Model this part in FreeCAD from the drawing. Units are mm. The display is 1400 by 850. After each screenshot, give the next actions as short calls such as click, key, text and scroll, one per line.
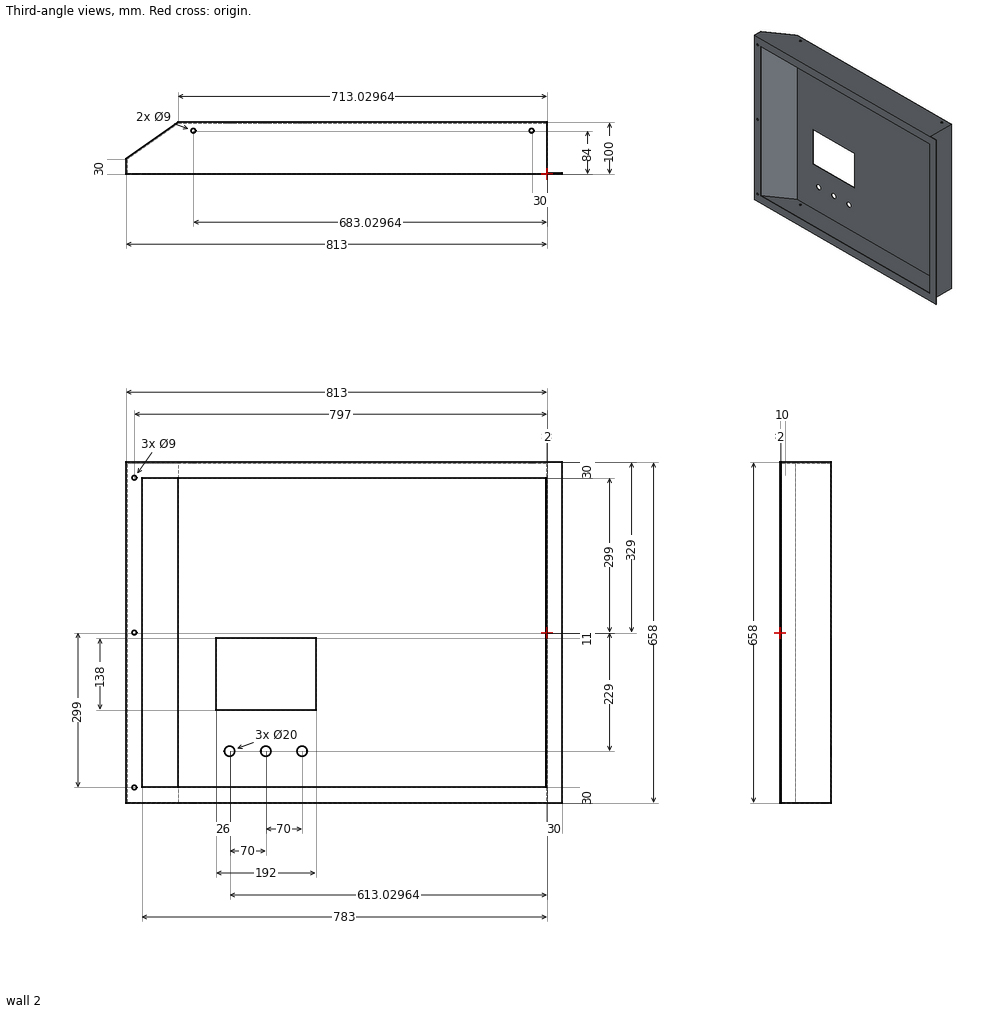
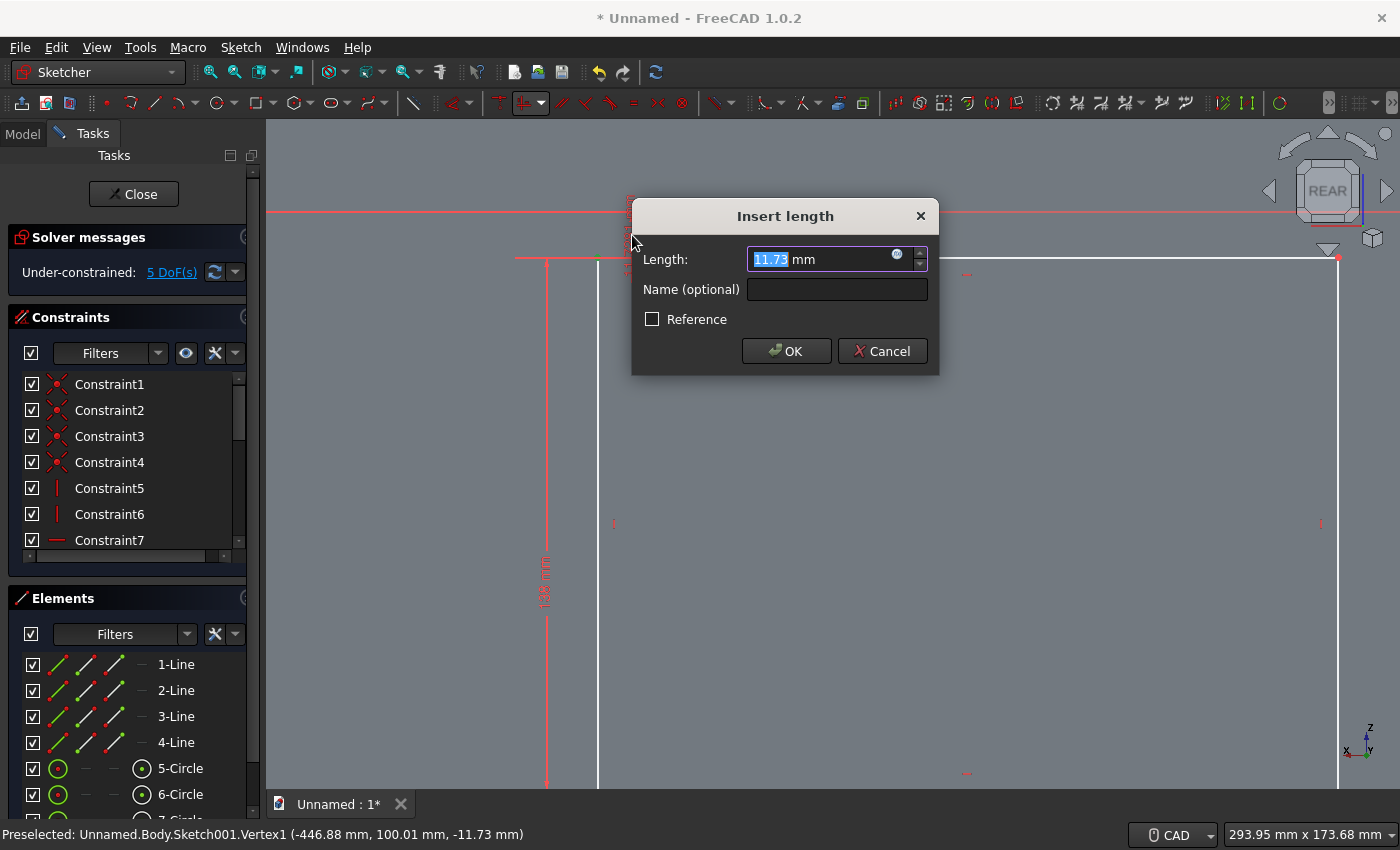
text(11)
key(Return)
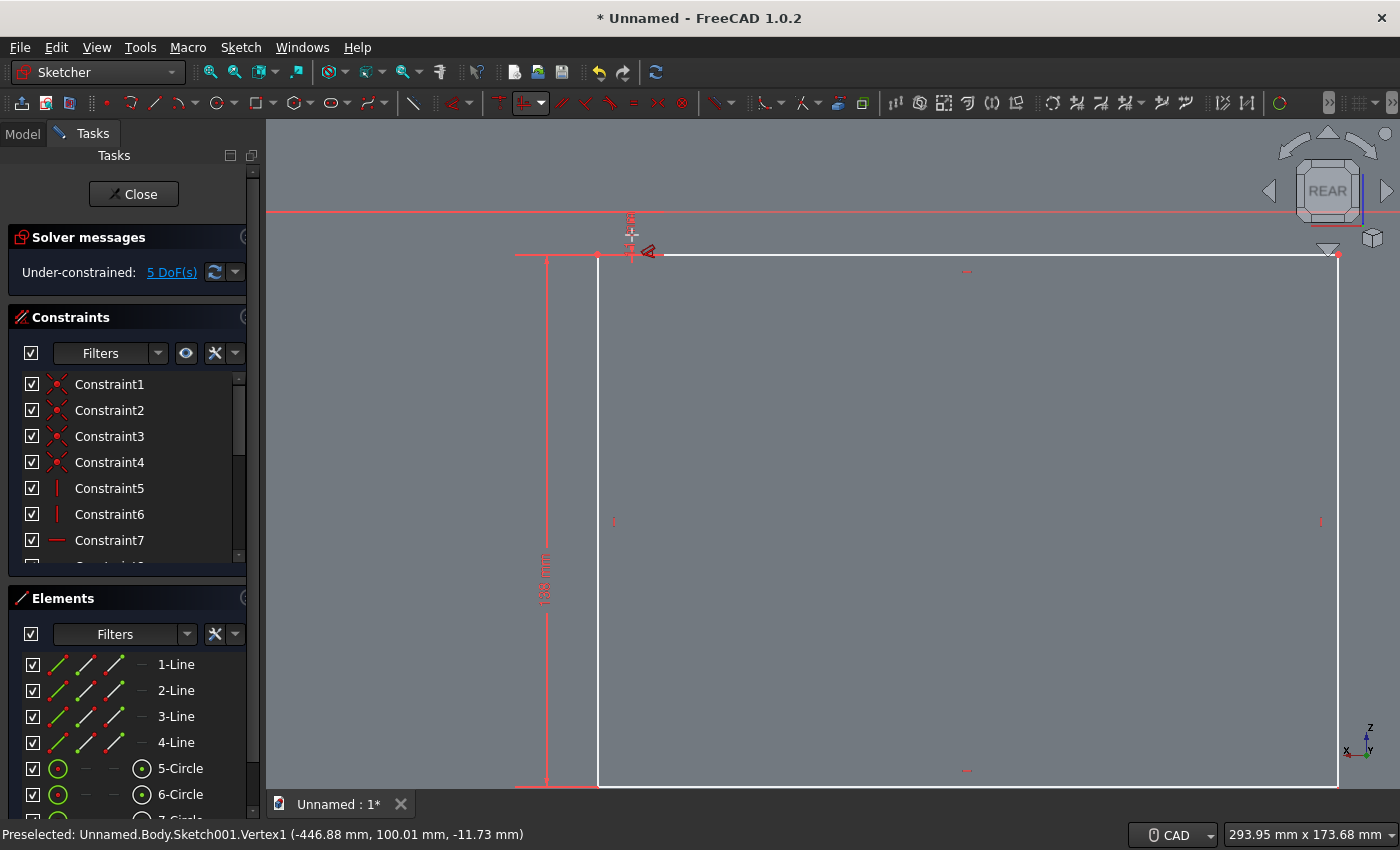
scroll(598, 258, down, 4)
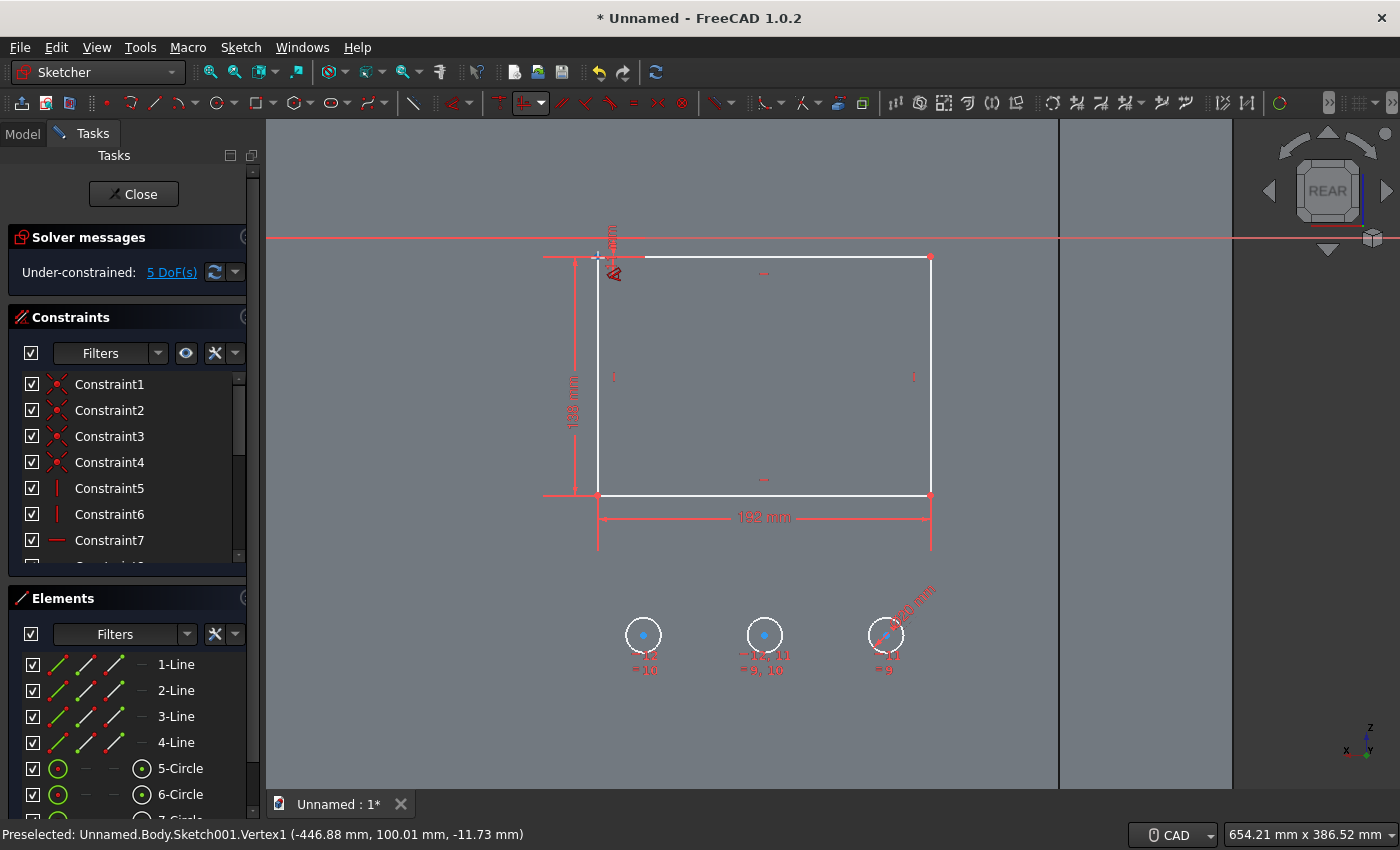
click(886, 635)
click(920, 528)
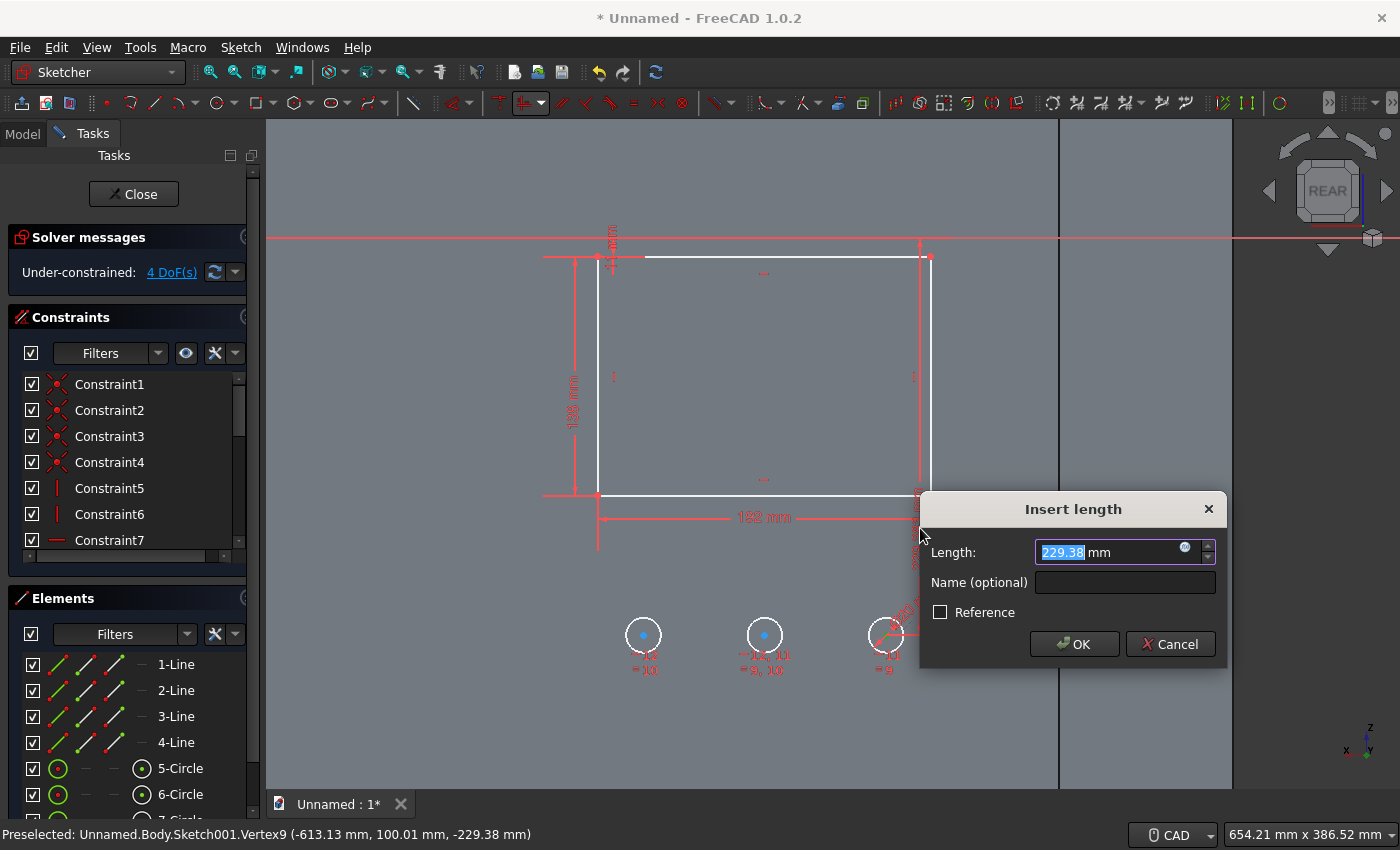
text(229)
key(Return)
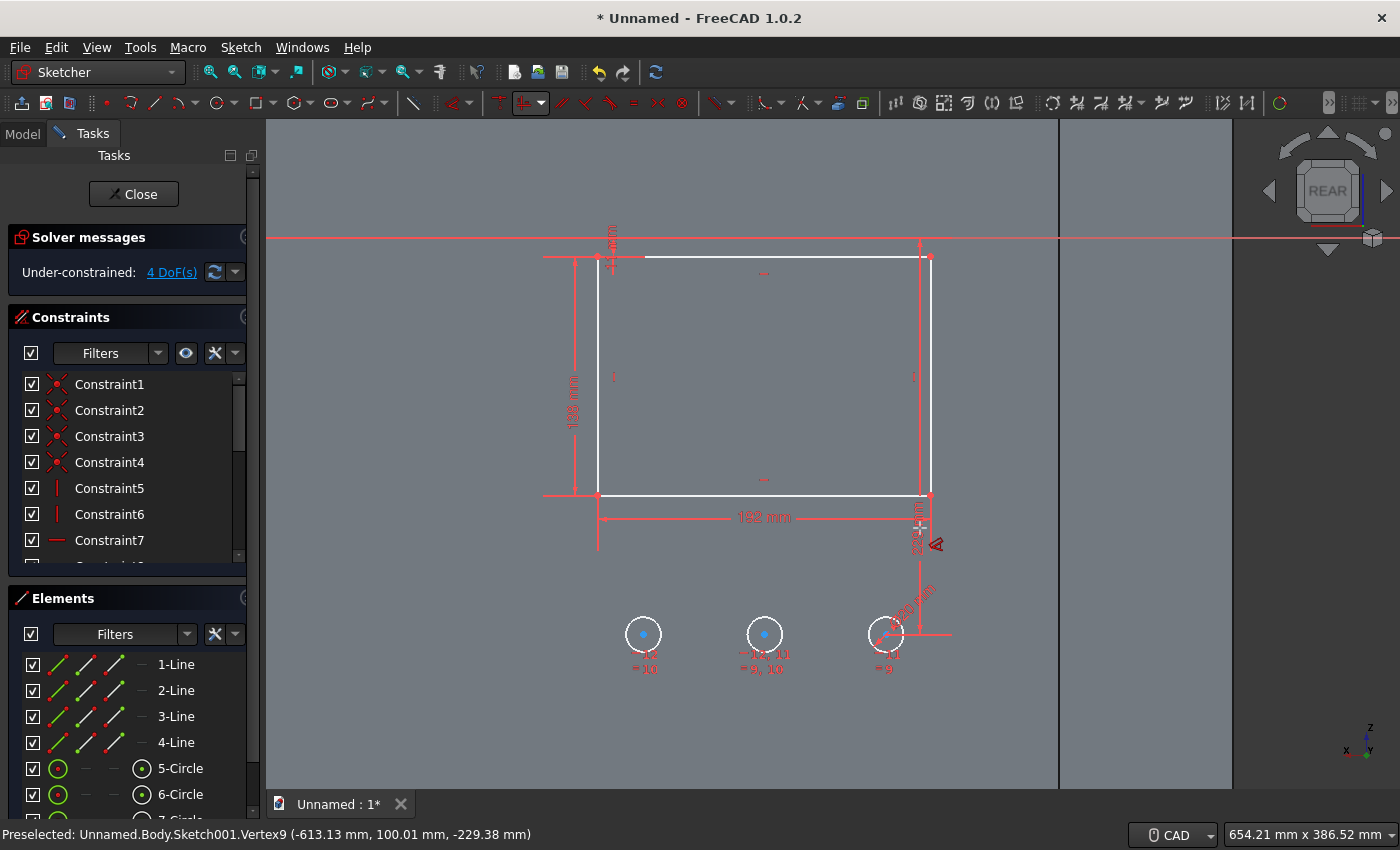
click(931, 496)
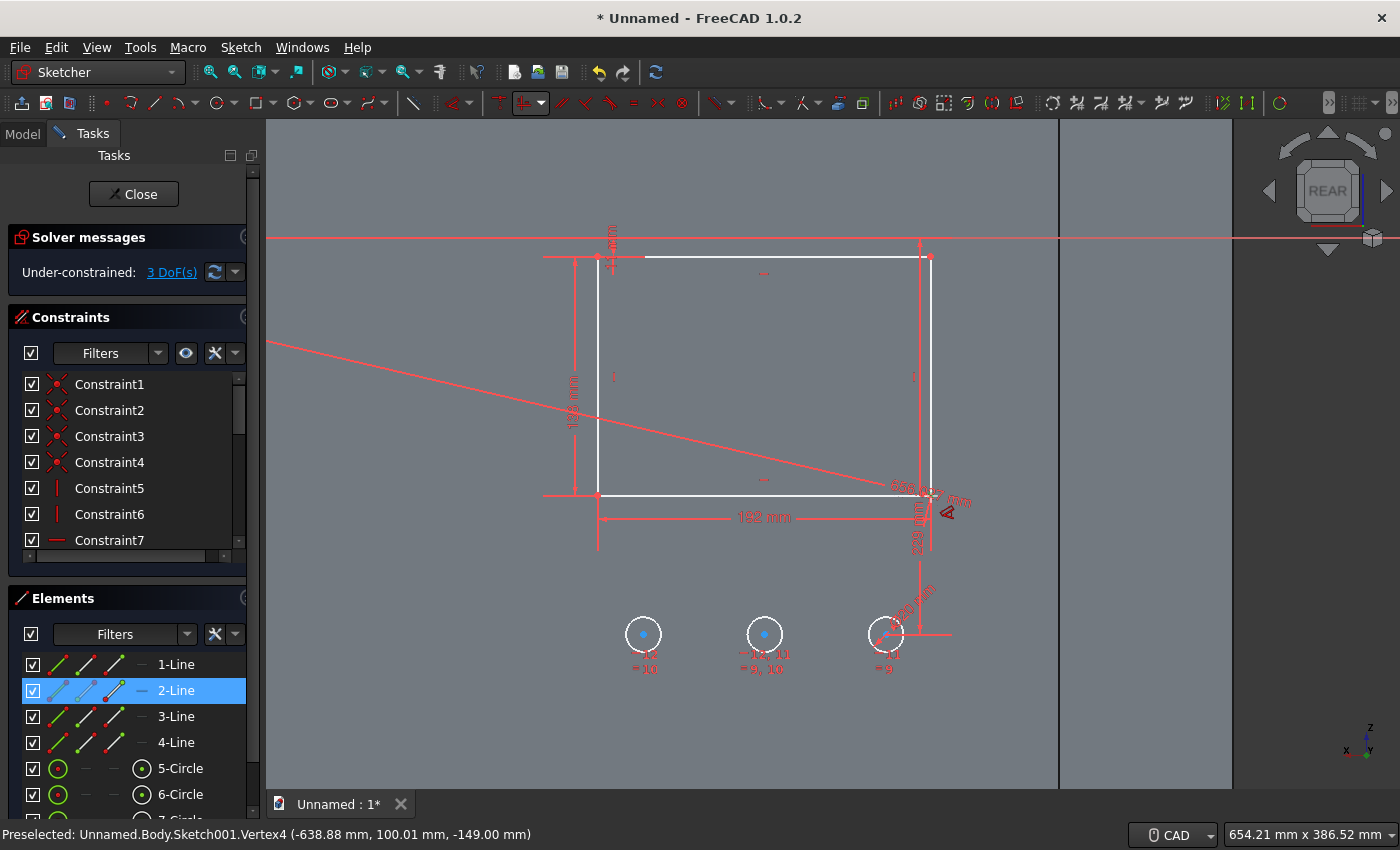
click(886, 635)
click(908, 669)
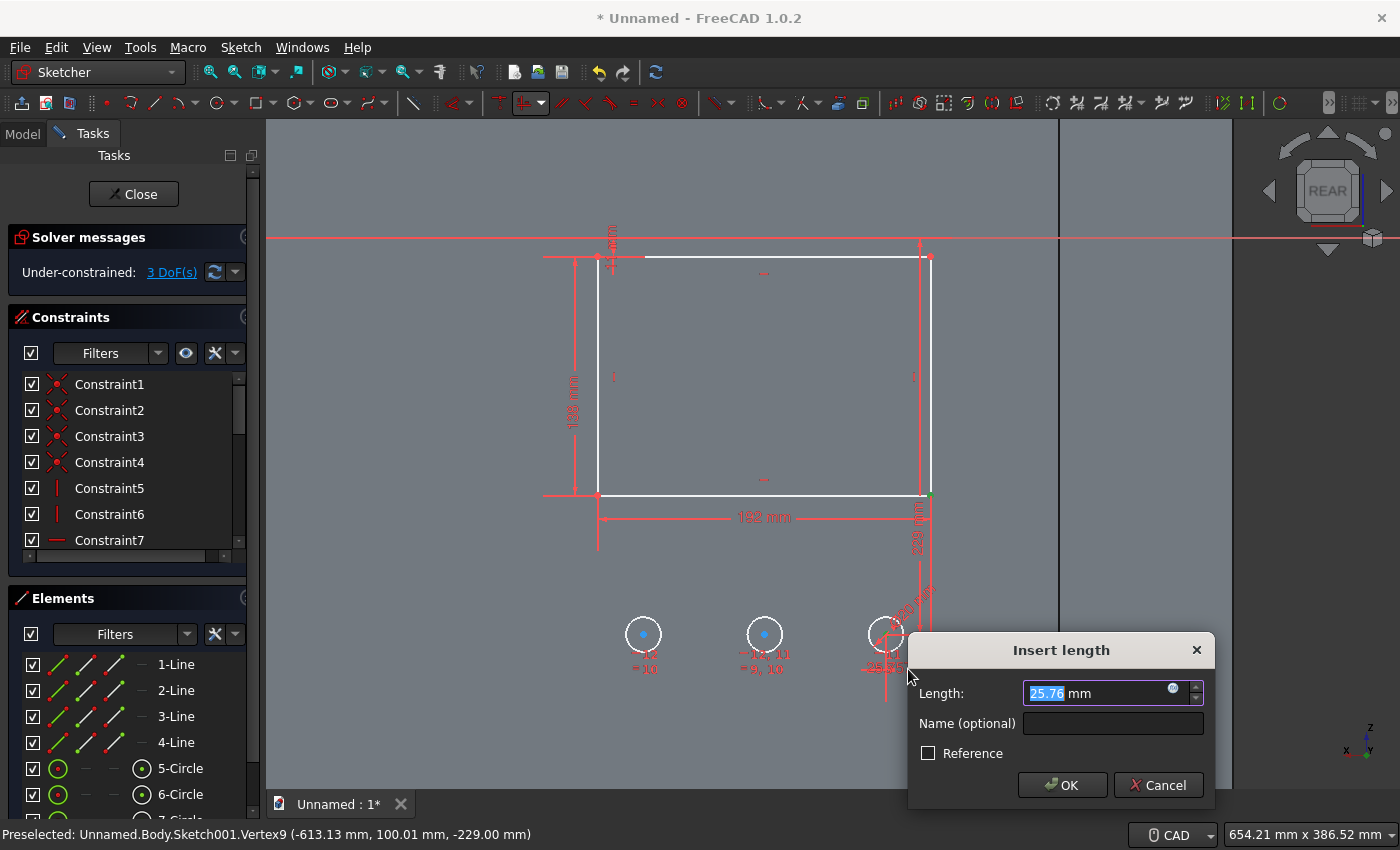
text(26)
key(Return)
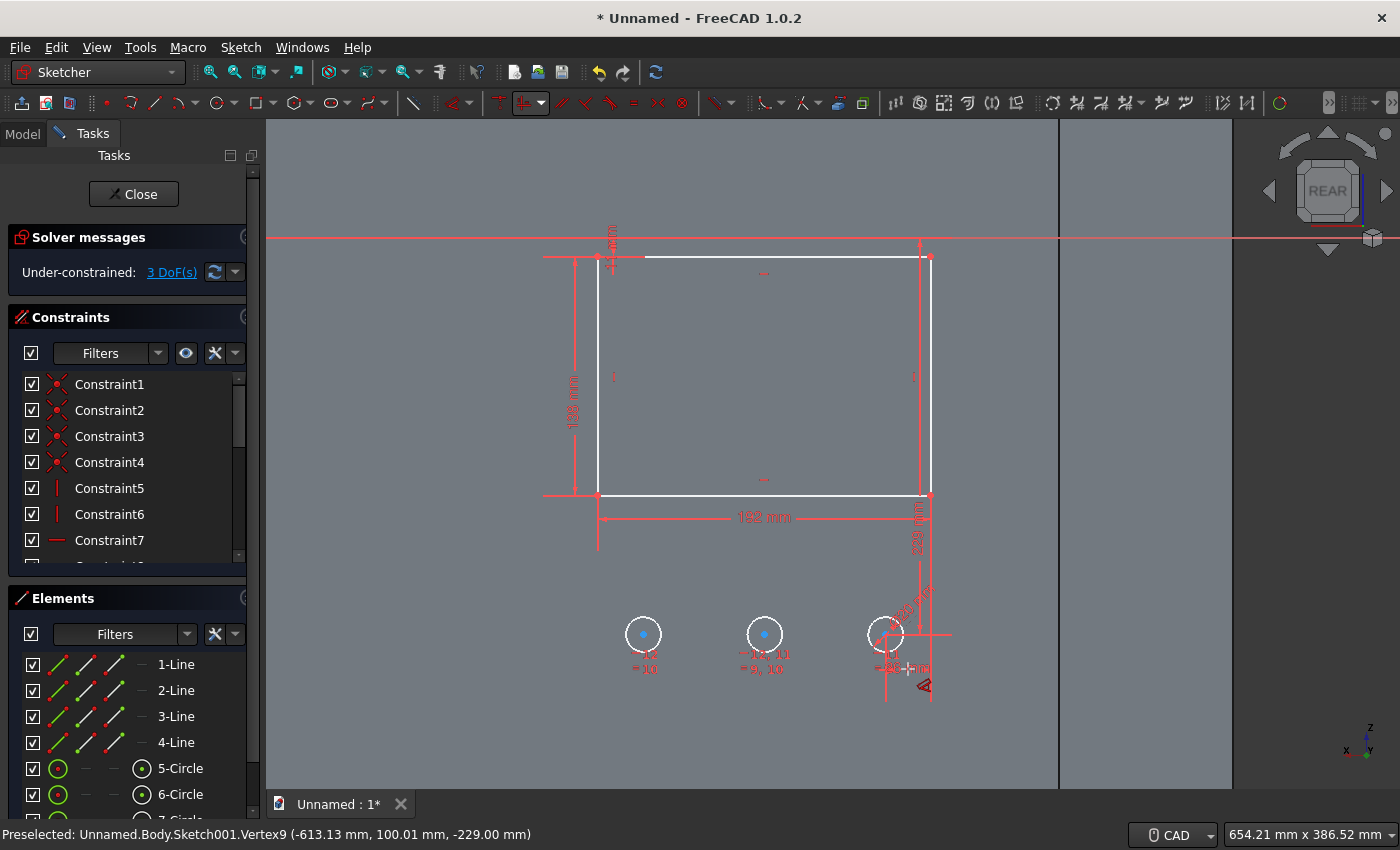
click(886, 635)